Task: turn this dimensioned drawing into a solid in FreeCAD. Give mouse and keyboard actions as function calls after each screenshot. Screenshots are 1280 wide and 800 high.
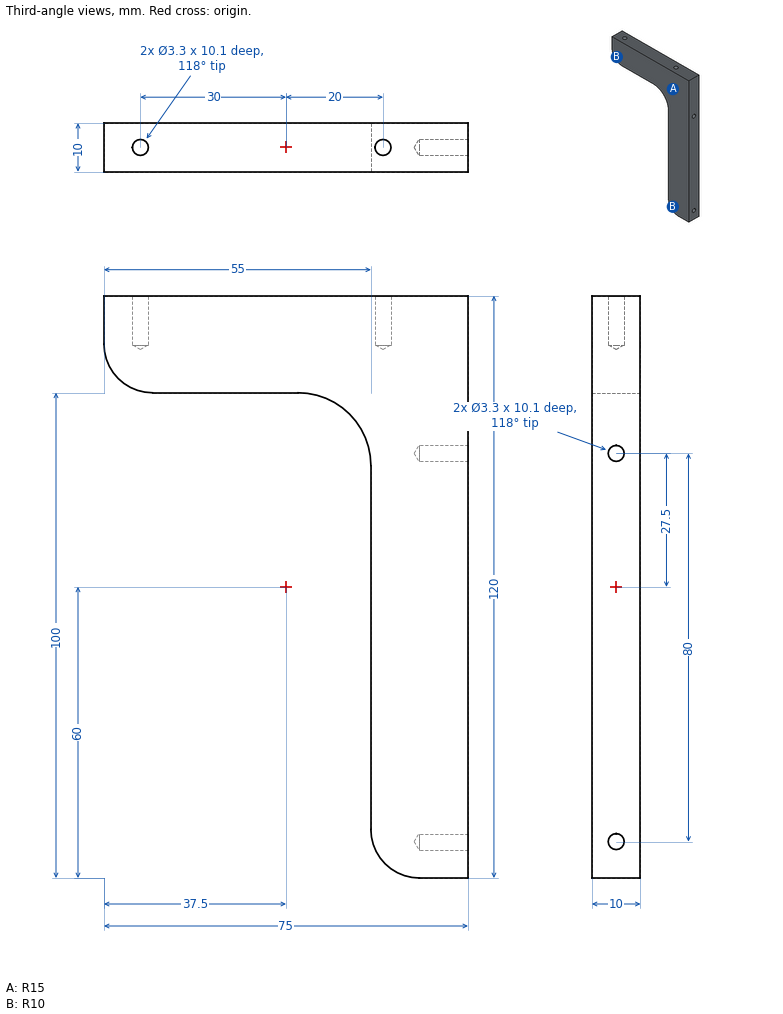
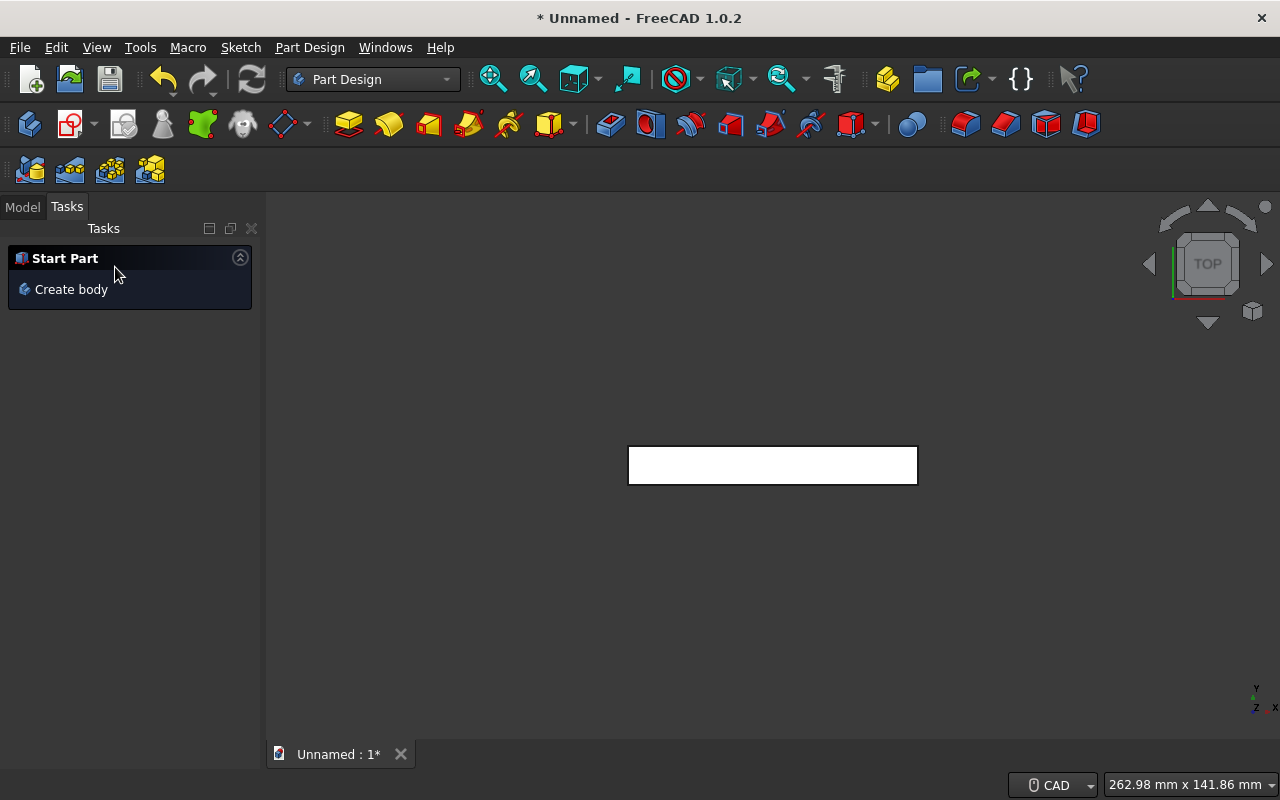
key(1)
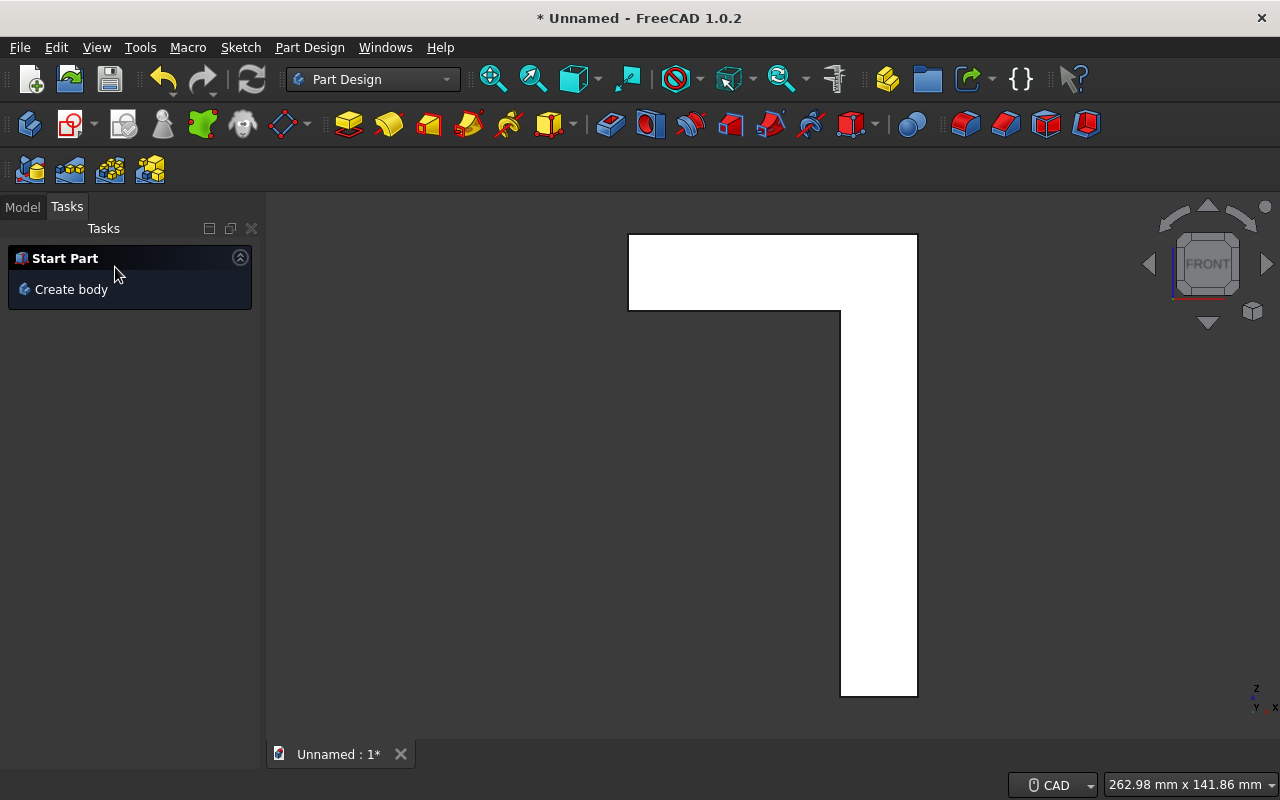
key(3)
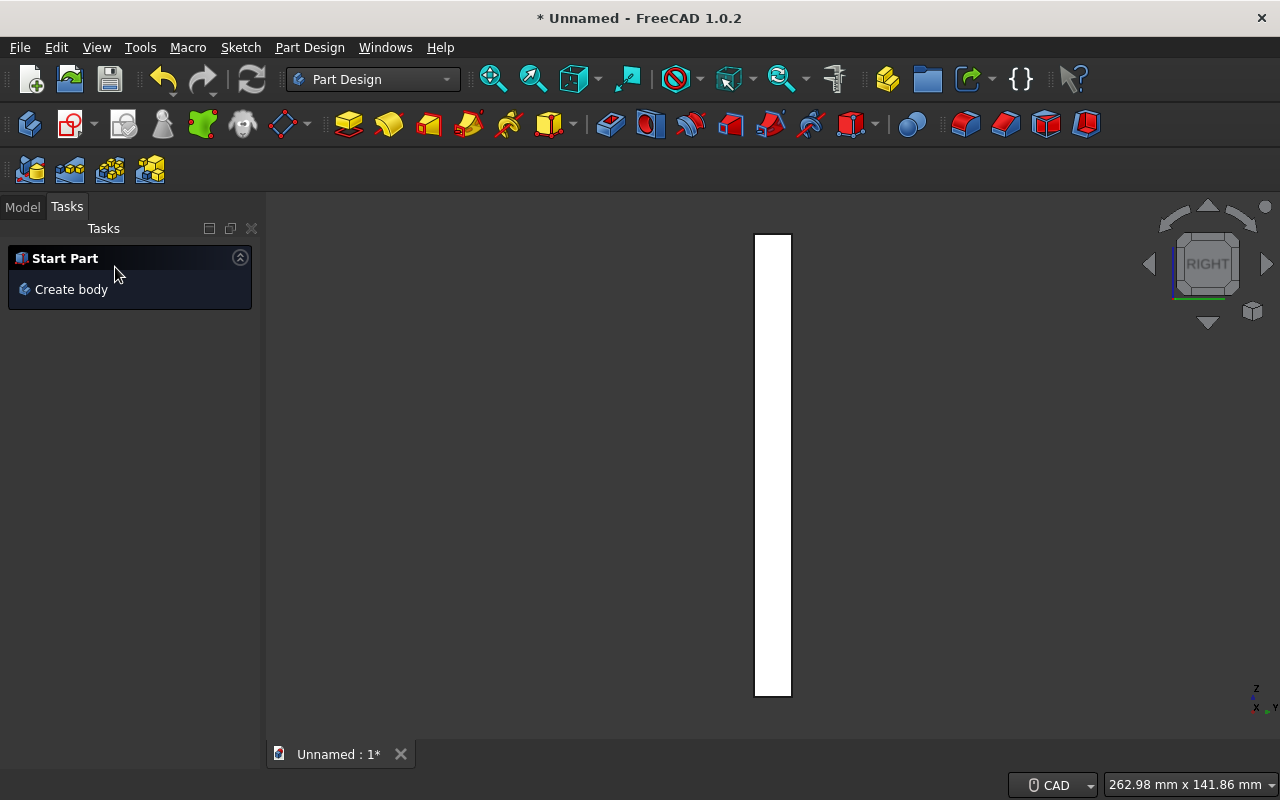
key(5)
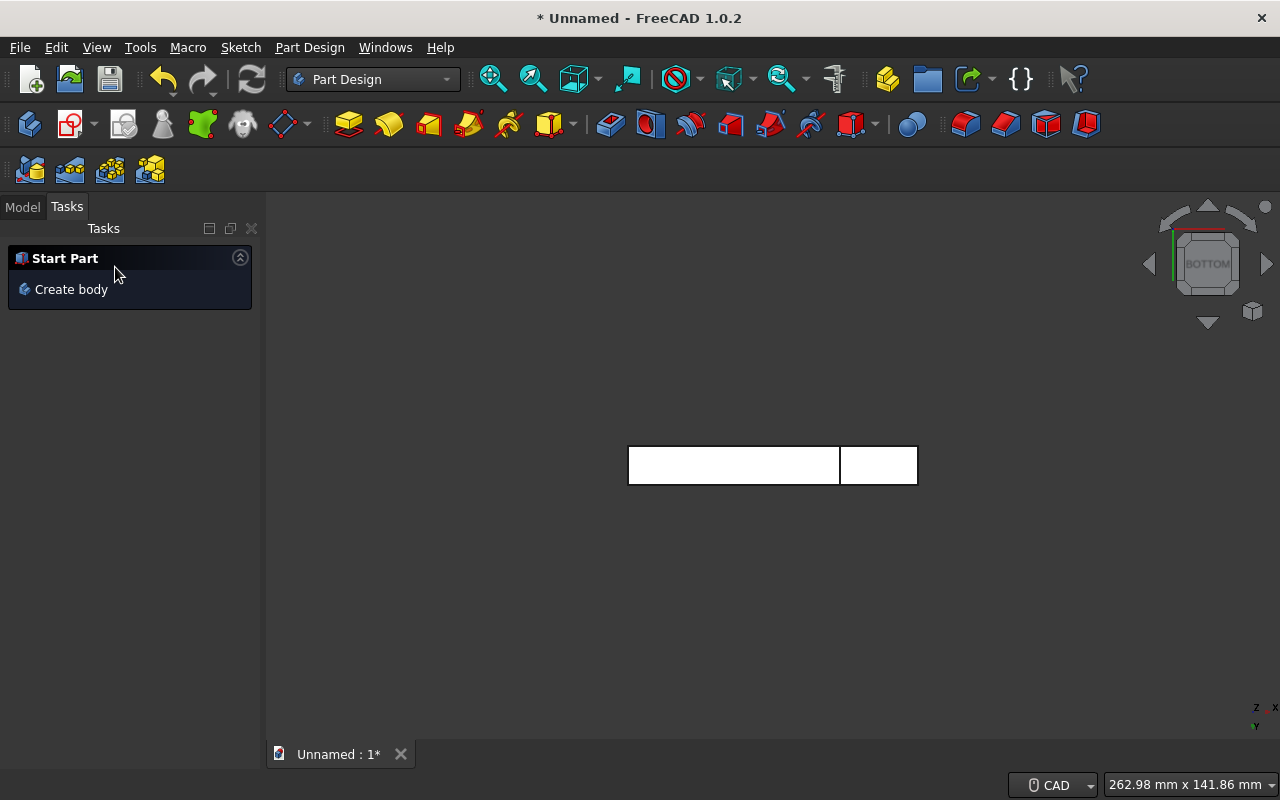
key(v)
key(f)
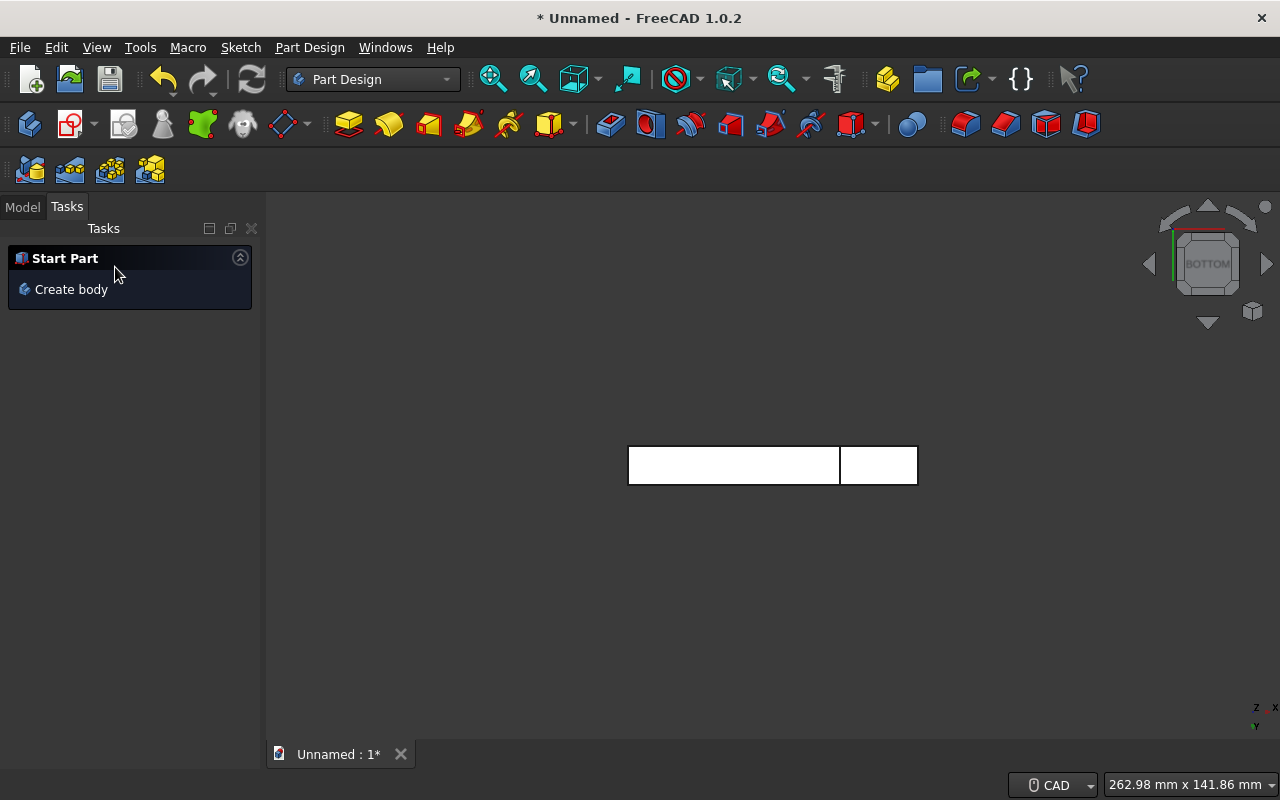
key(4)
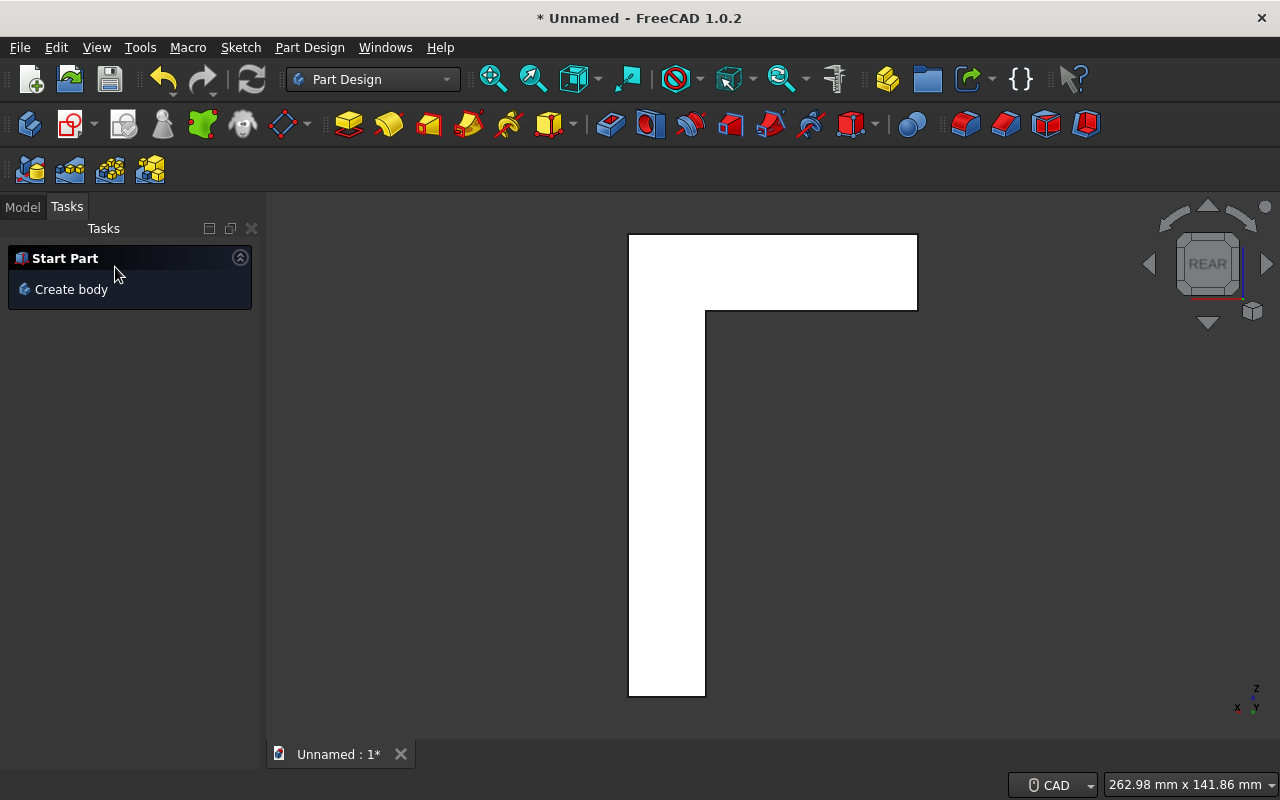
key(6)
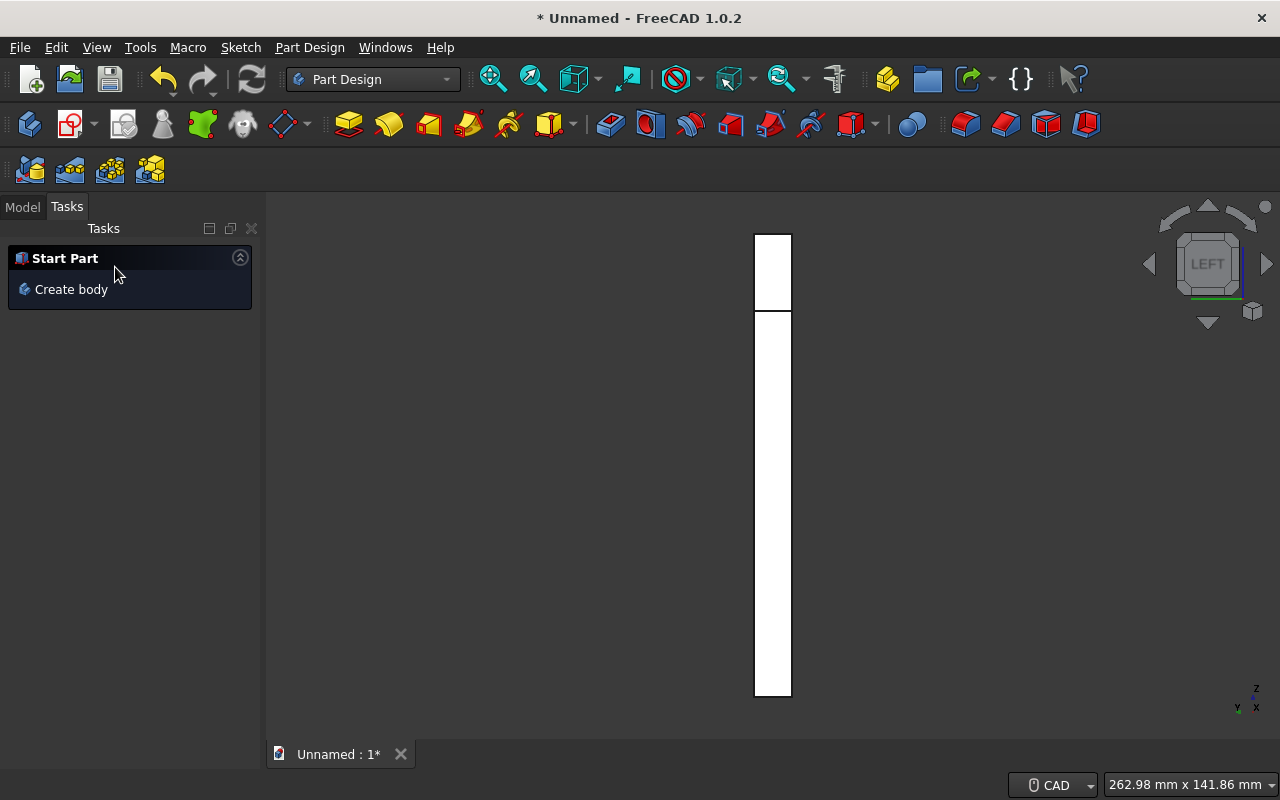
key(v)
key(3)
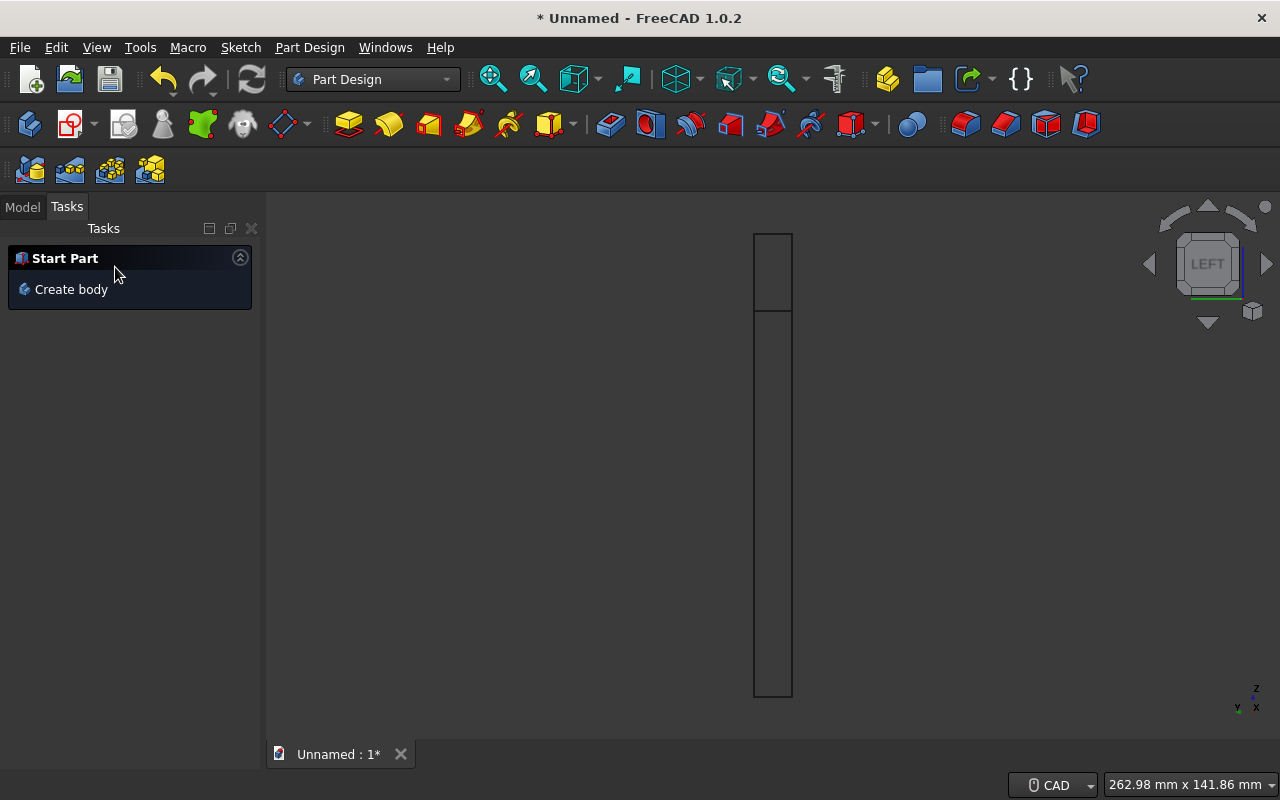
key(0)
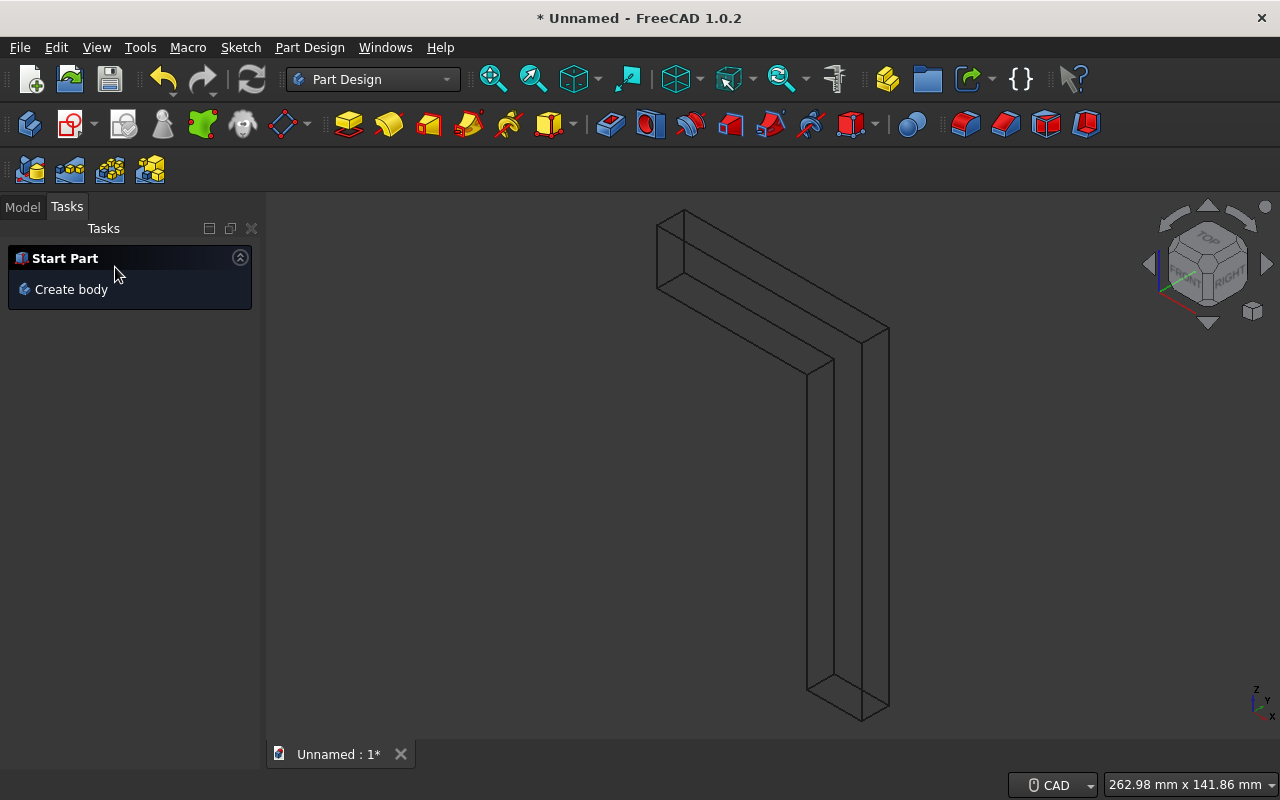
click(821, 366)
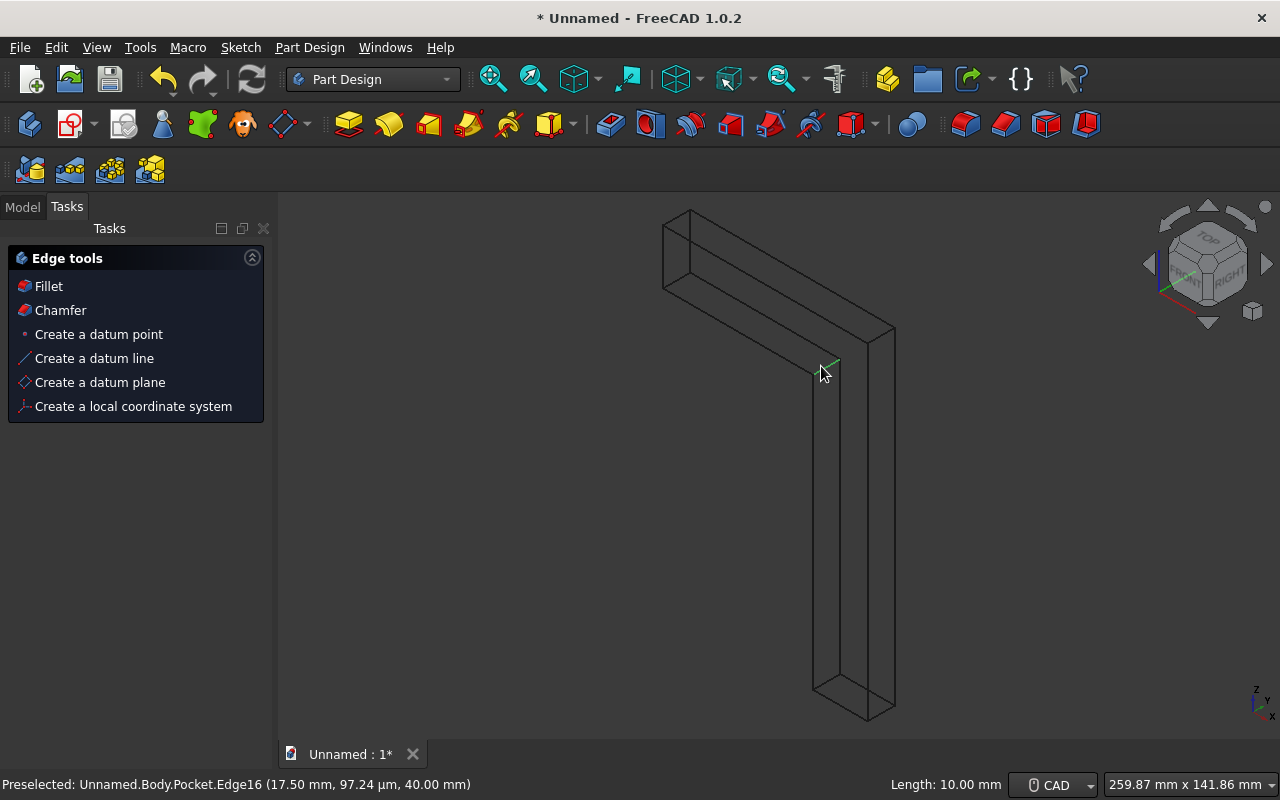
key(v)
key(1)